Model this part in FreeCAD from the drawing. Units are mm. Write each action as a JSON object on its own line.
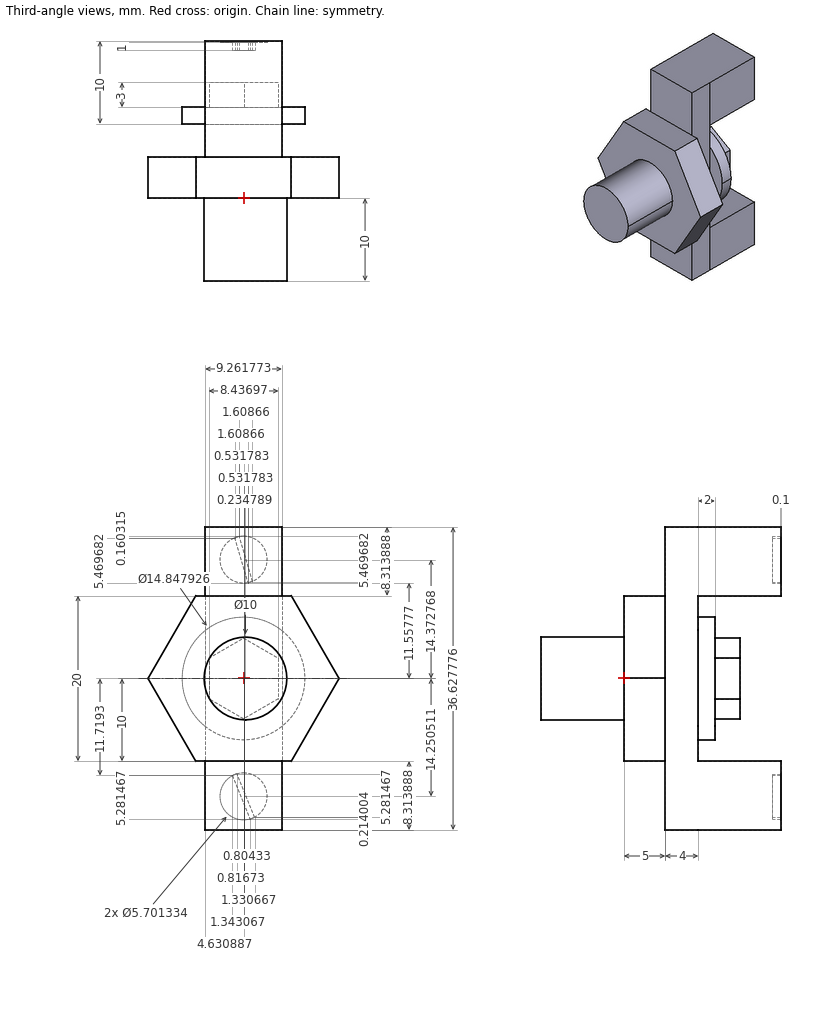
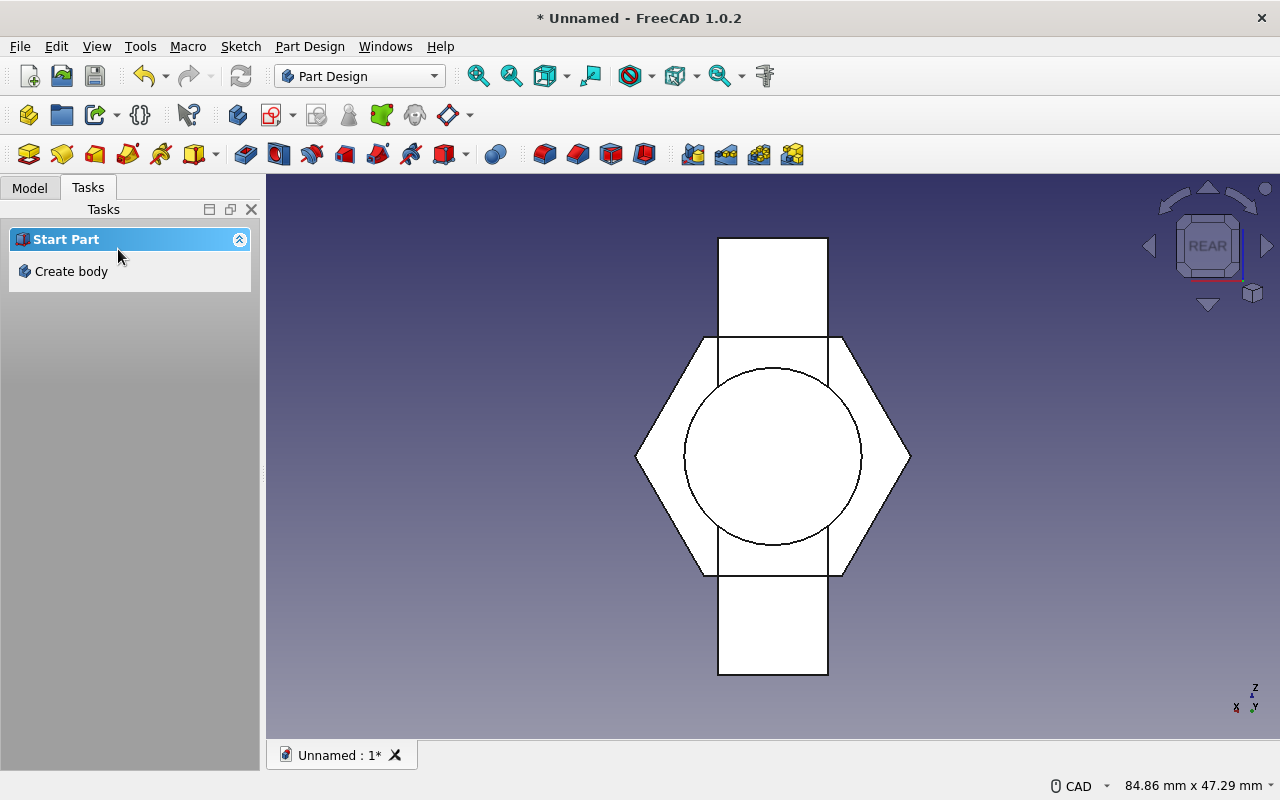
{"action": "left_click", "coordinate": [773, 455]}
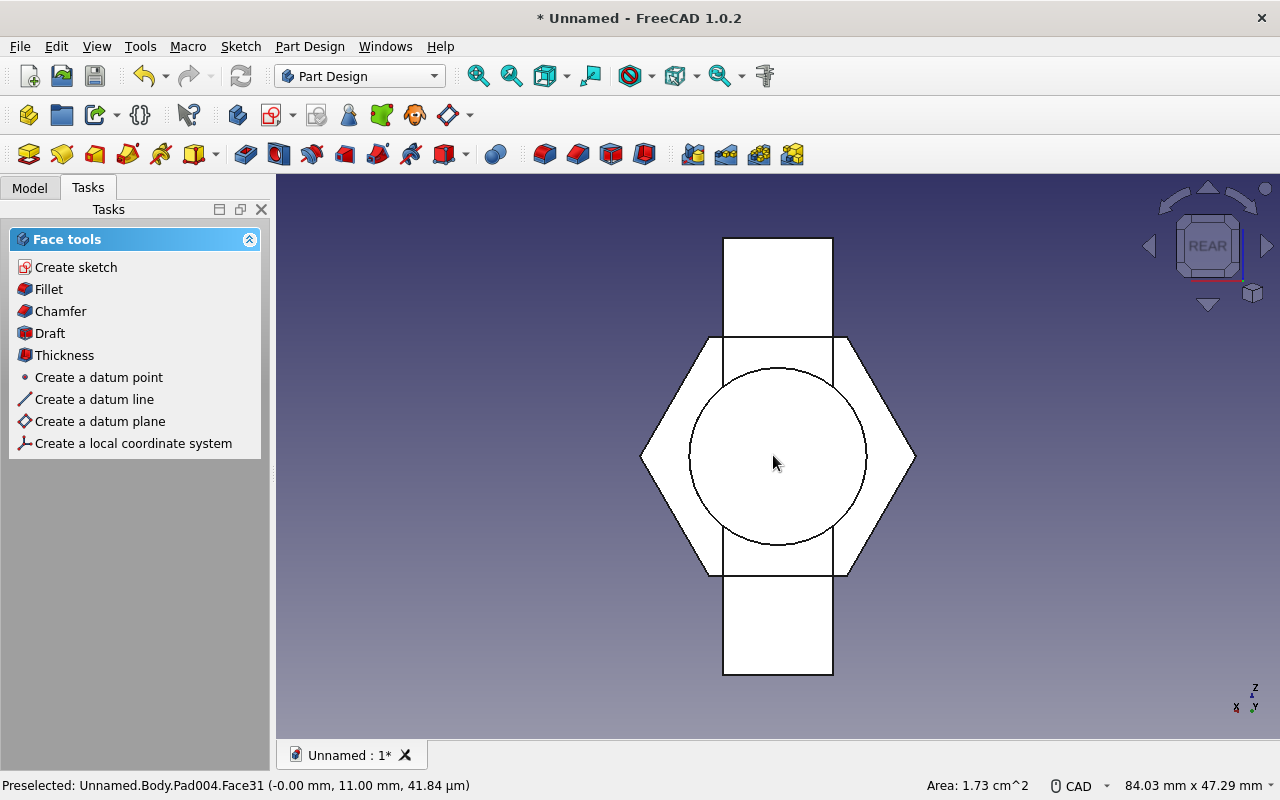
{"action": "left_click", "coordinate": [270, 116]}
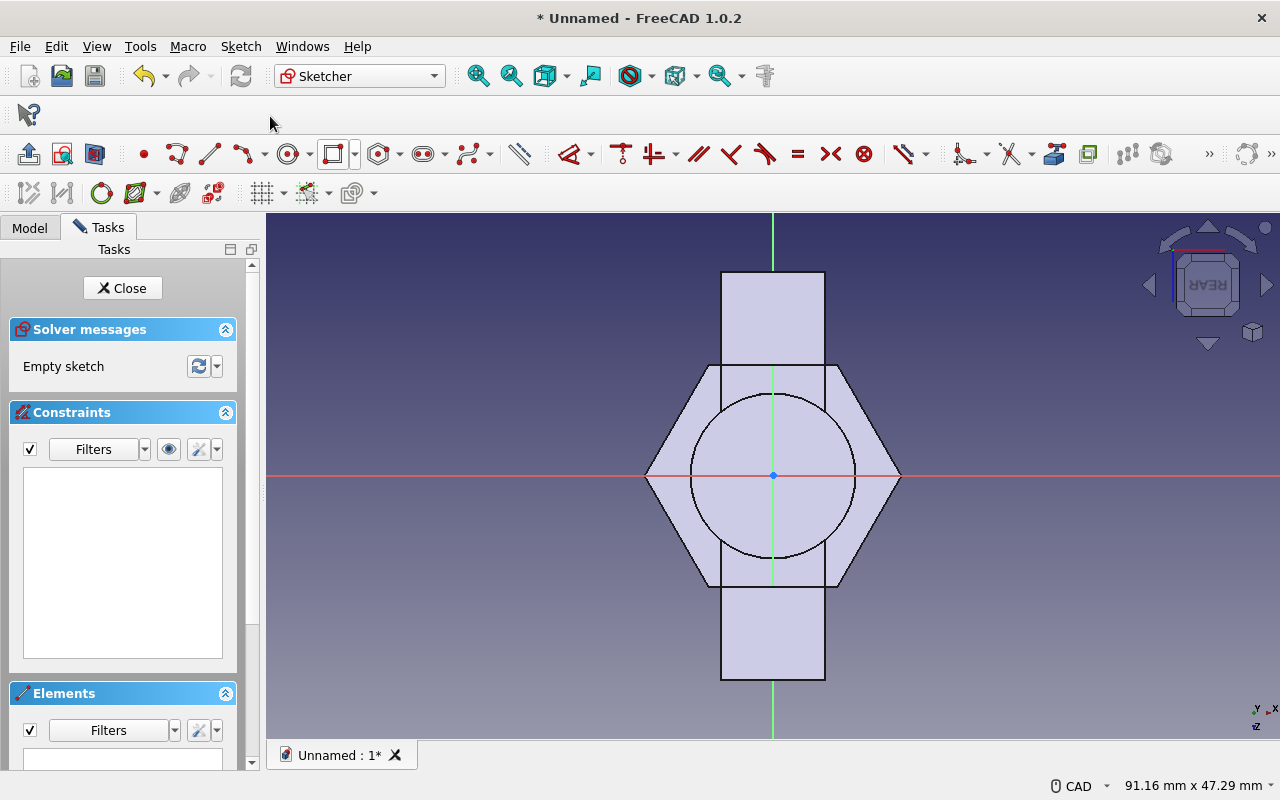
{"action": "scroll", "coordinate": [803, 476], "scroll_direction": "up", "scroll_amount": 6}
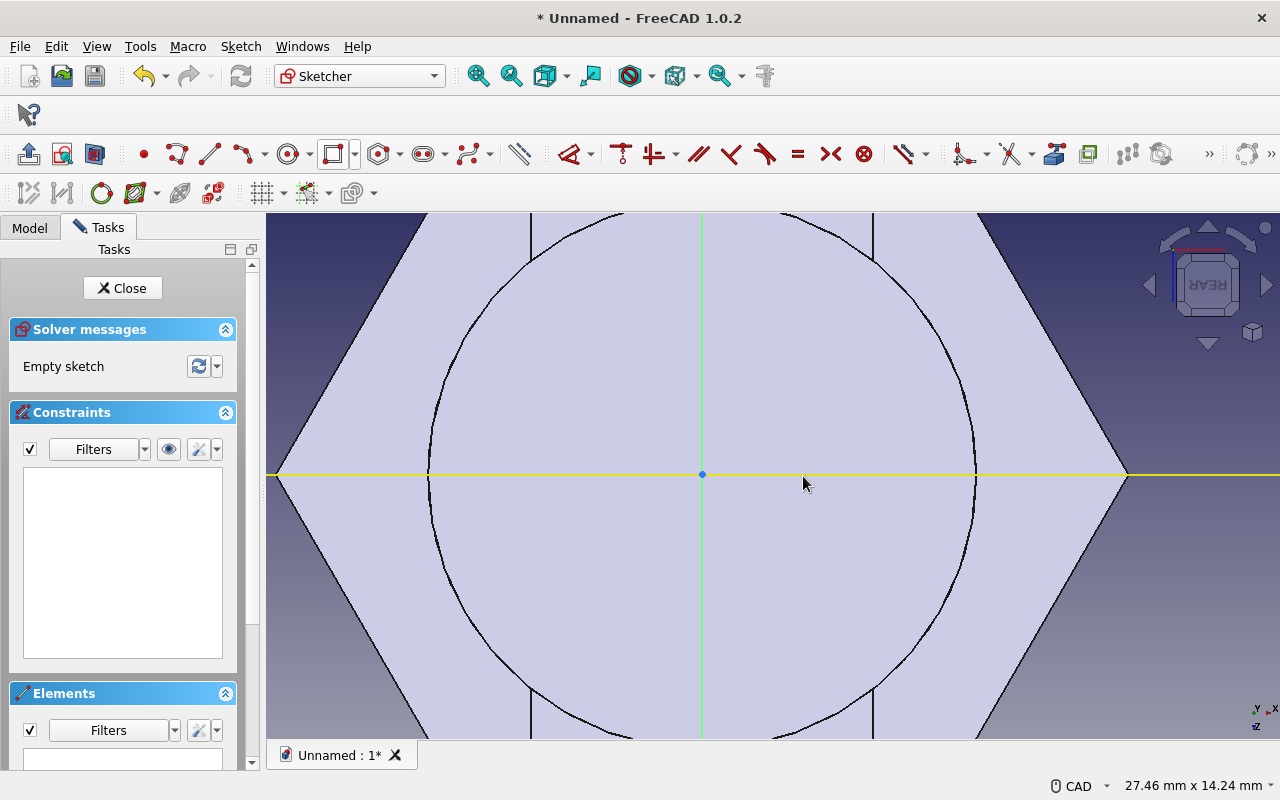
{"action": "left_click", "coordinate": [378, 154]}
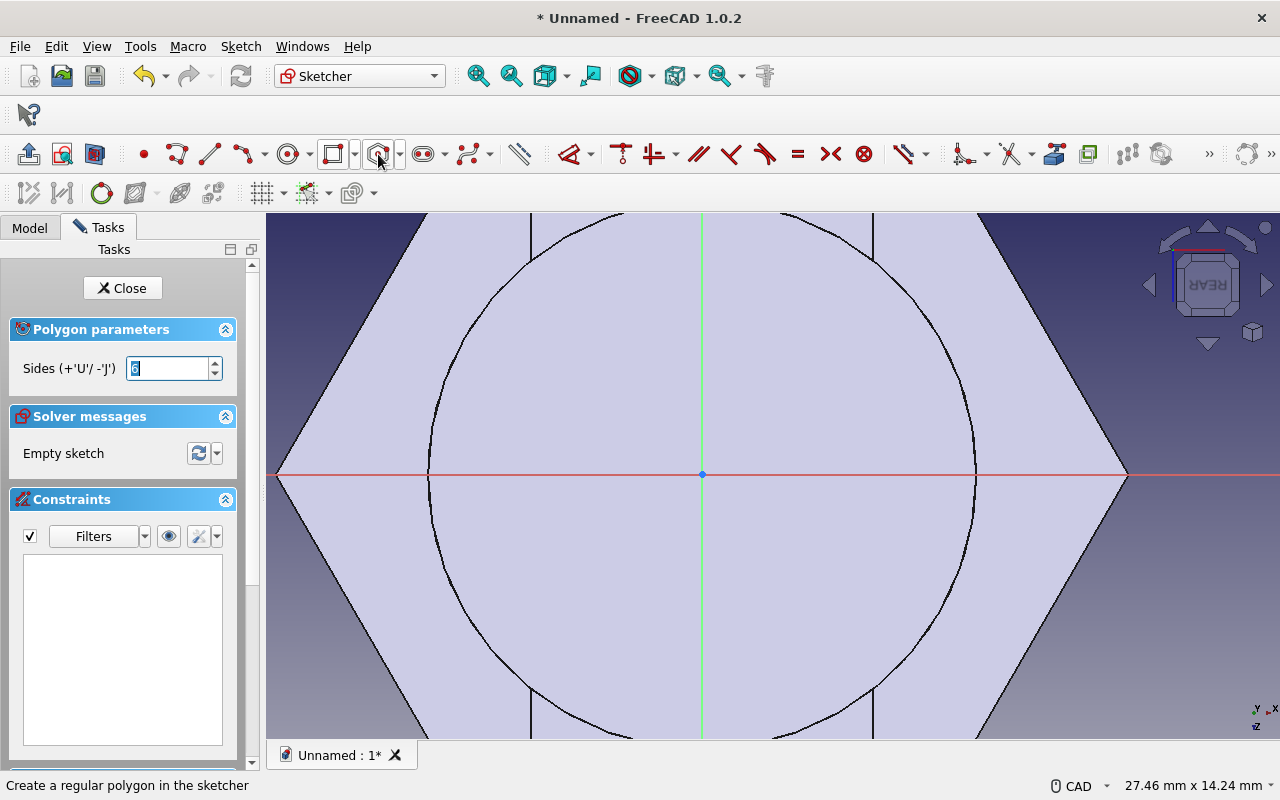
{"action": "left_click", "coordinate": [702, 475]}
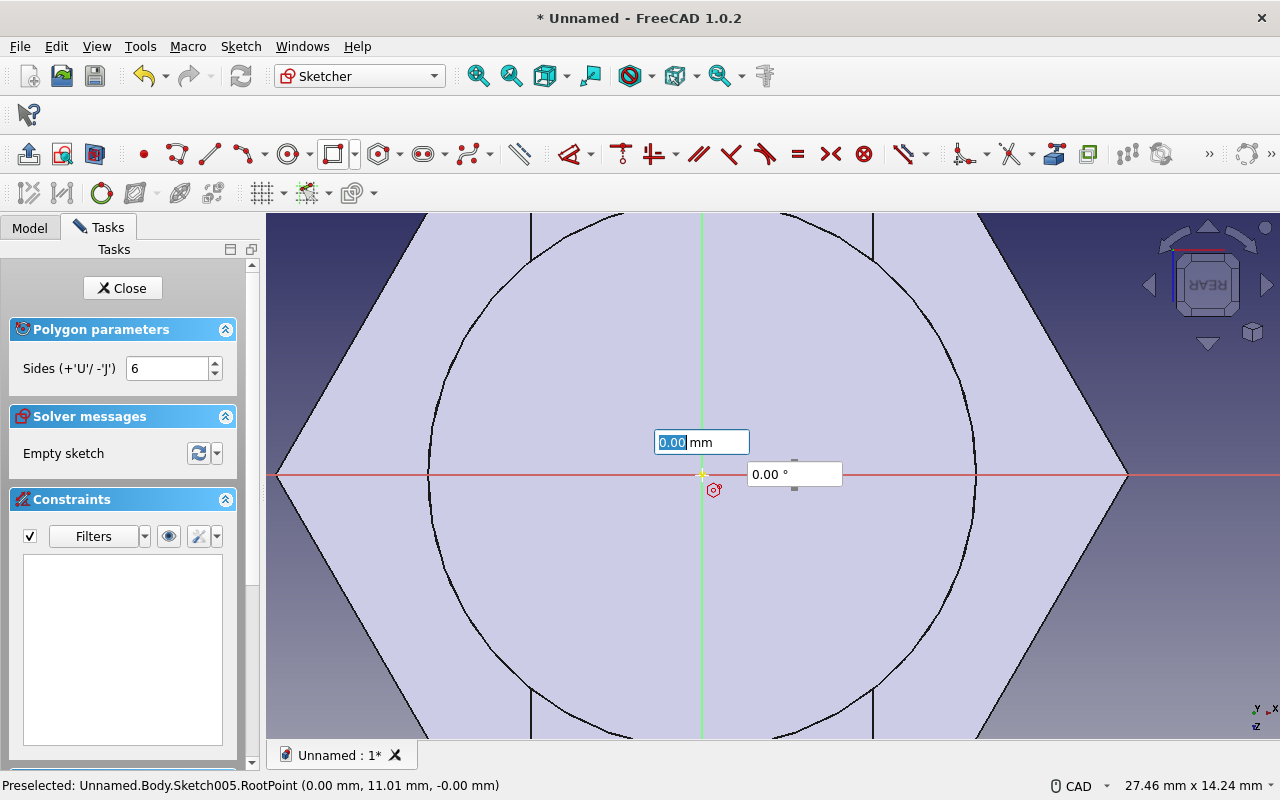
{"action": "left_click", "coordinate": [702, 295]}
{"action": "key", "text": "Escape"}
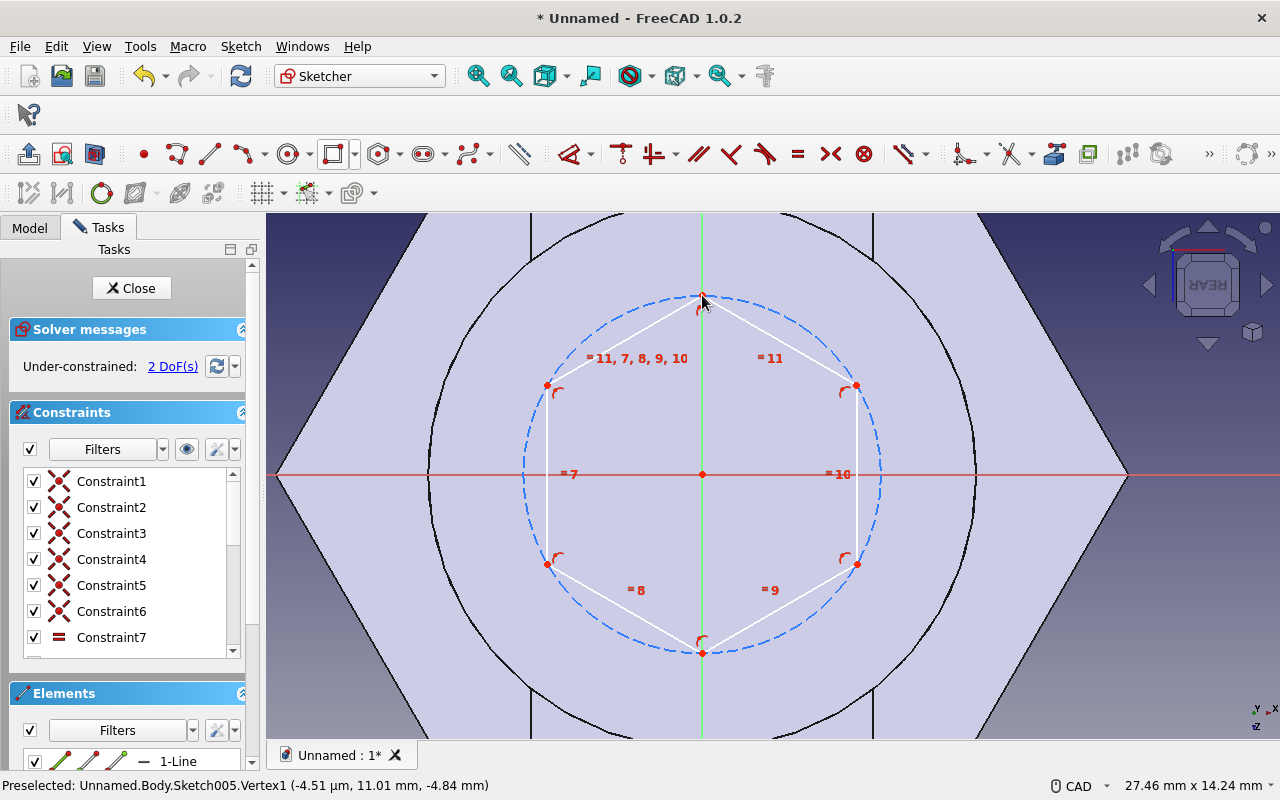
{"action": "left_click", "coordinate": [547, 439]}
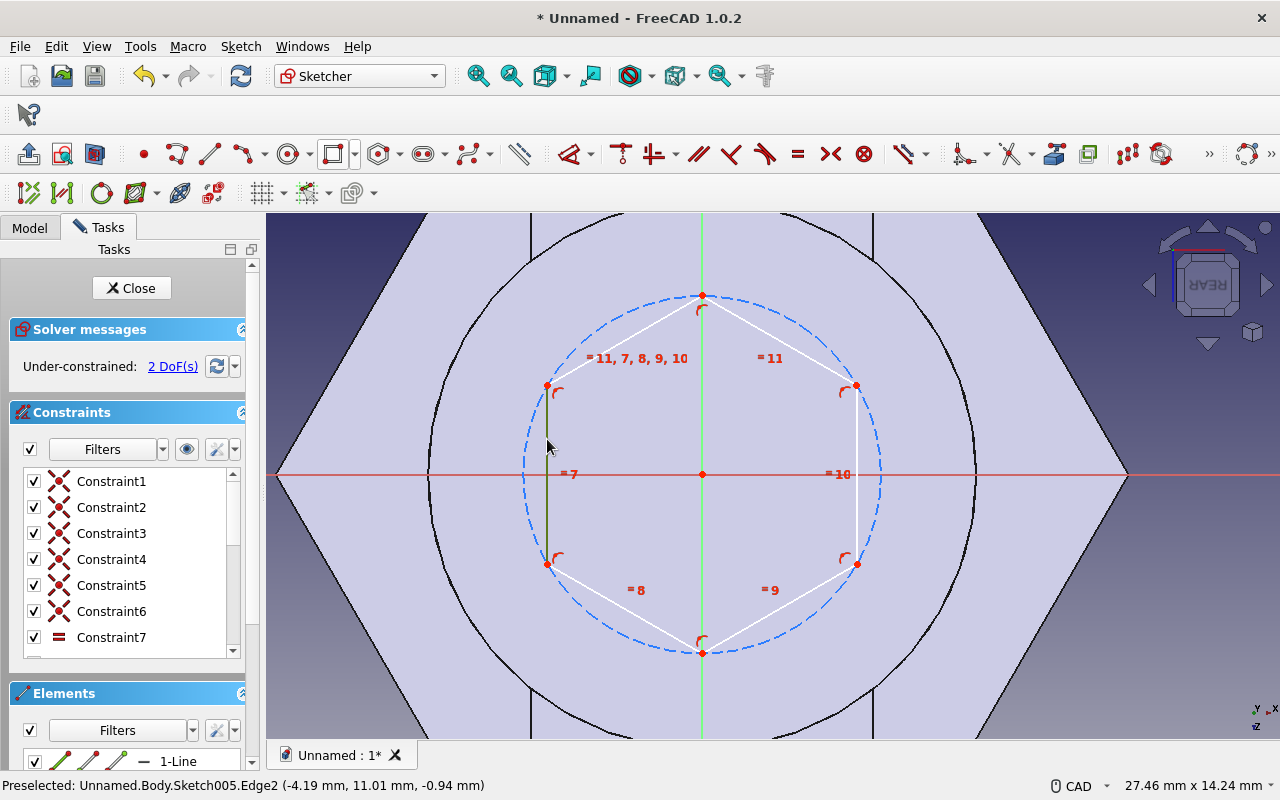
{"action": "left_click", "coordinate": [676, 154]}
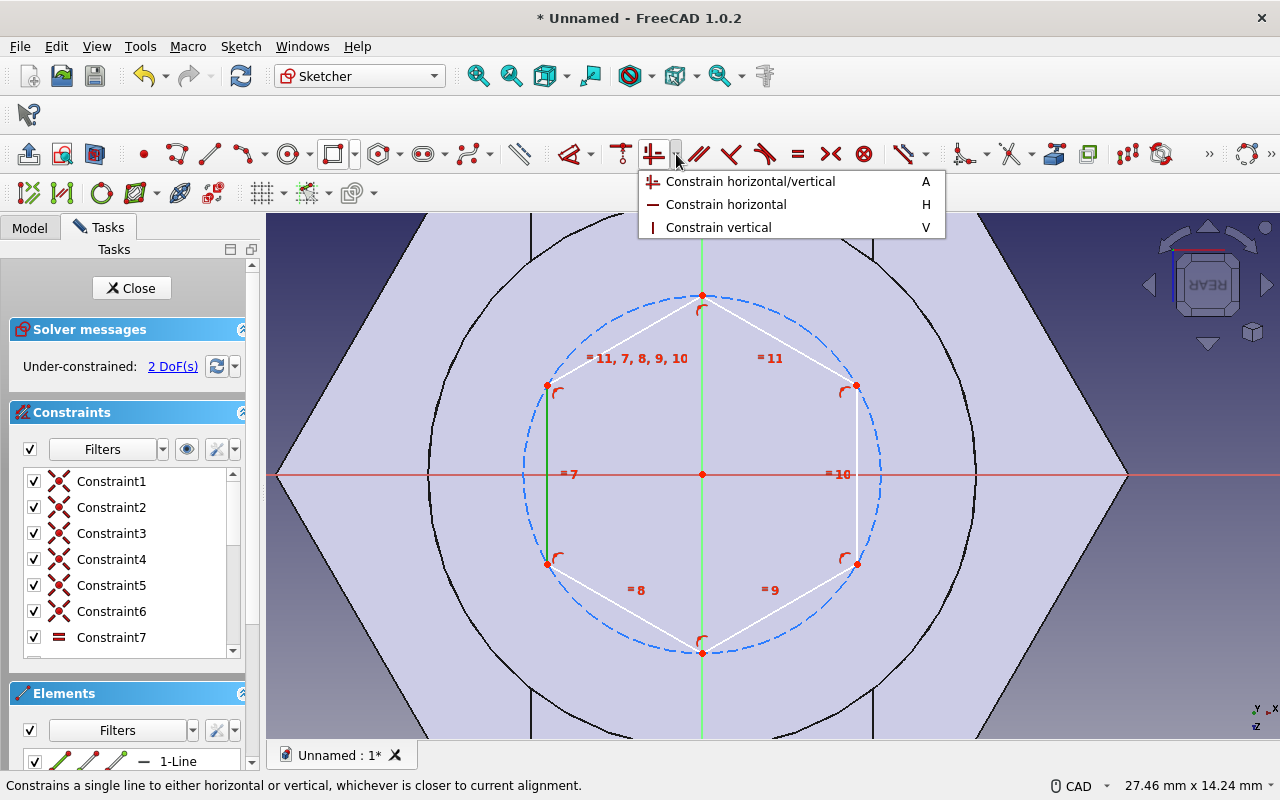
{"action": "left_click", "coordinate": [792, 228]}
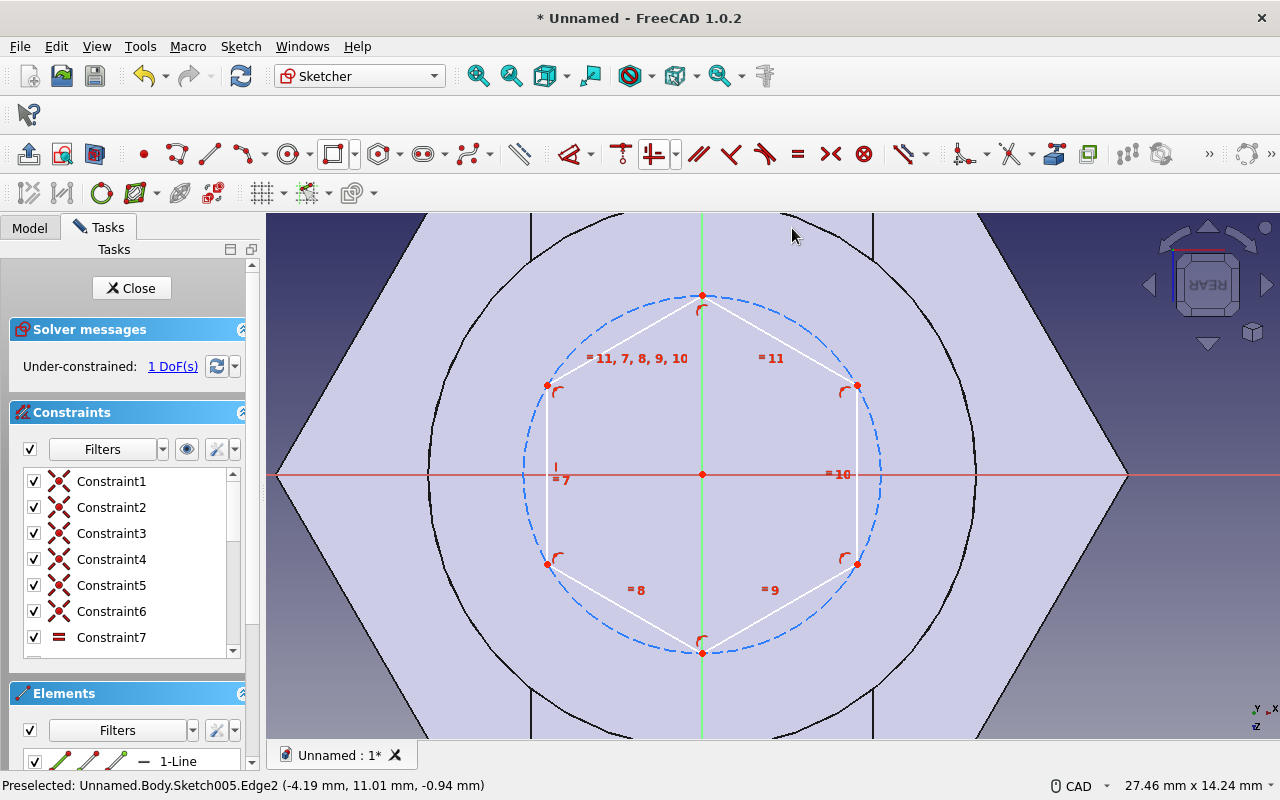
{"action": "left_click", "coordinate": [568, 154]}